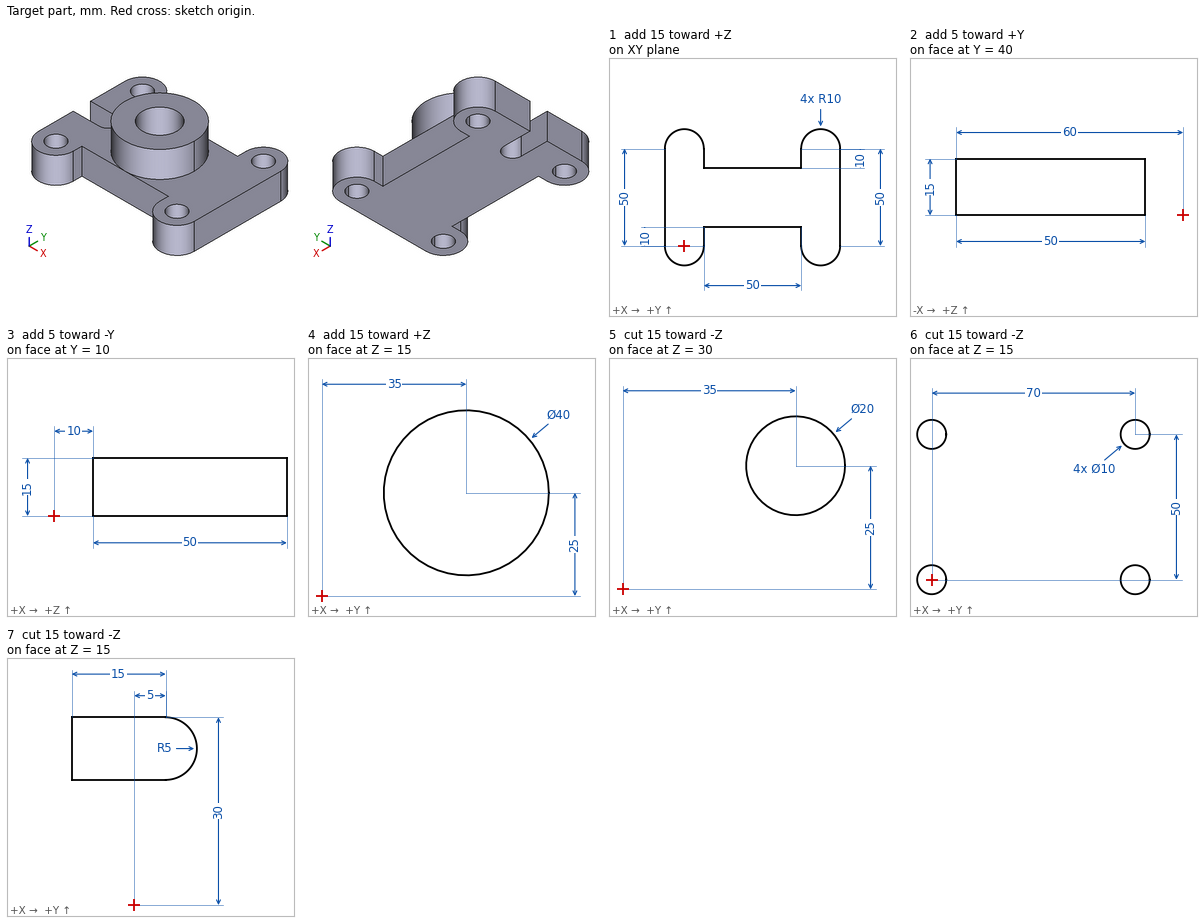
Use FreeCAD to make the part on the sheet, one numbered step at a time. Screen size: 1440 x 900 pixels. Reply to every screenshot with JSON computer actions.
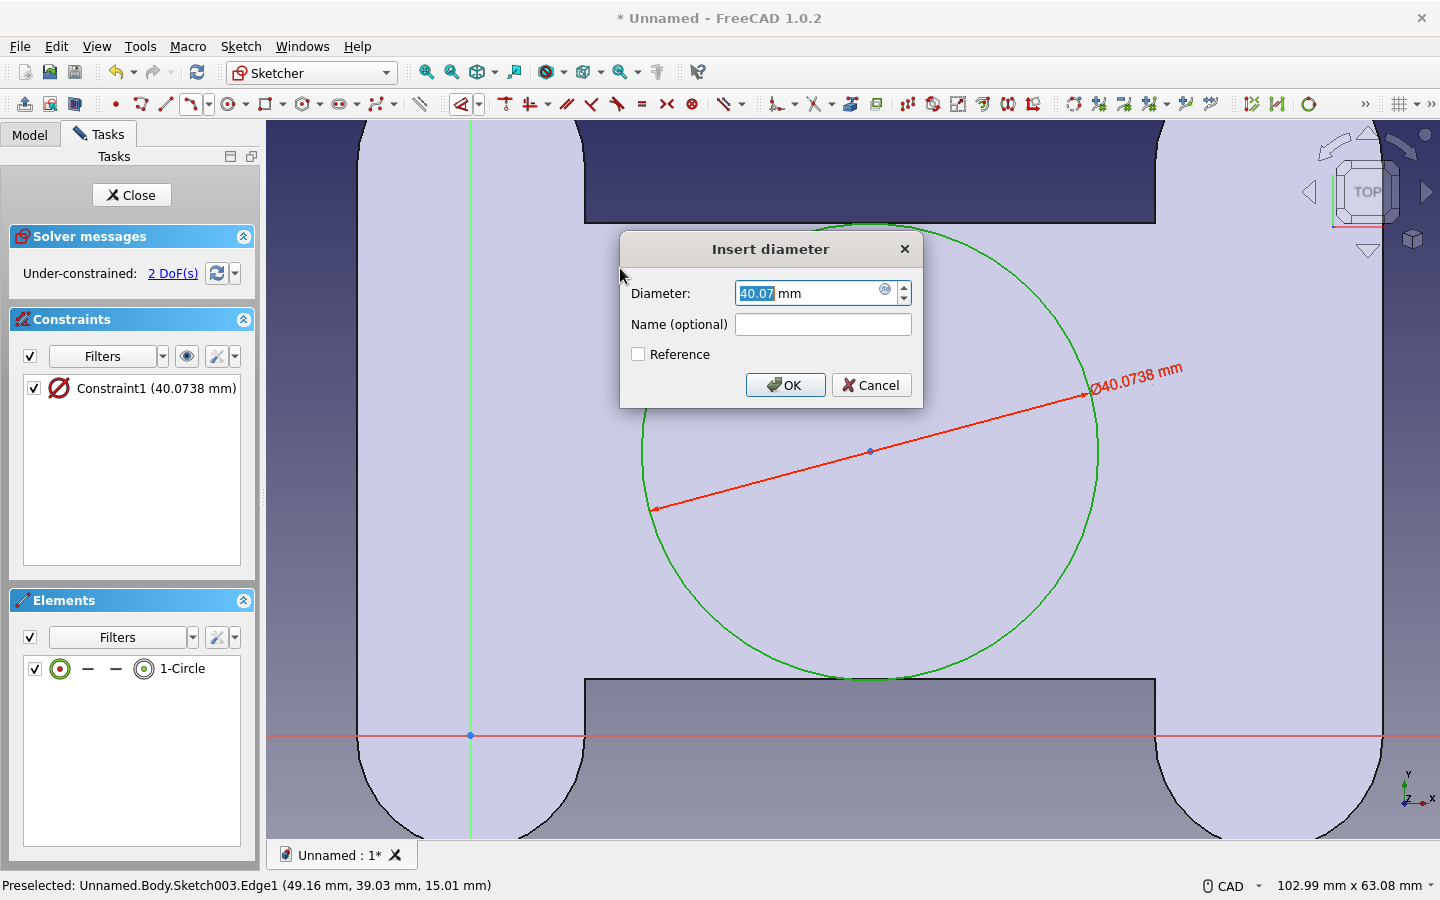
{"action": "type", "text": "40"}
{"action": "key", "text": "Return"}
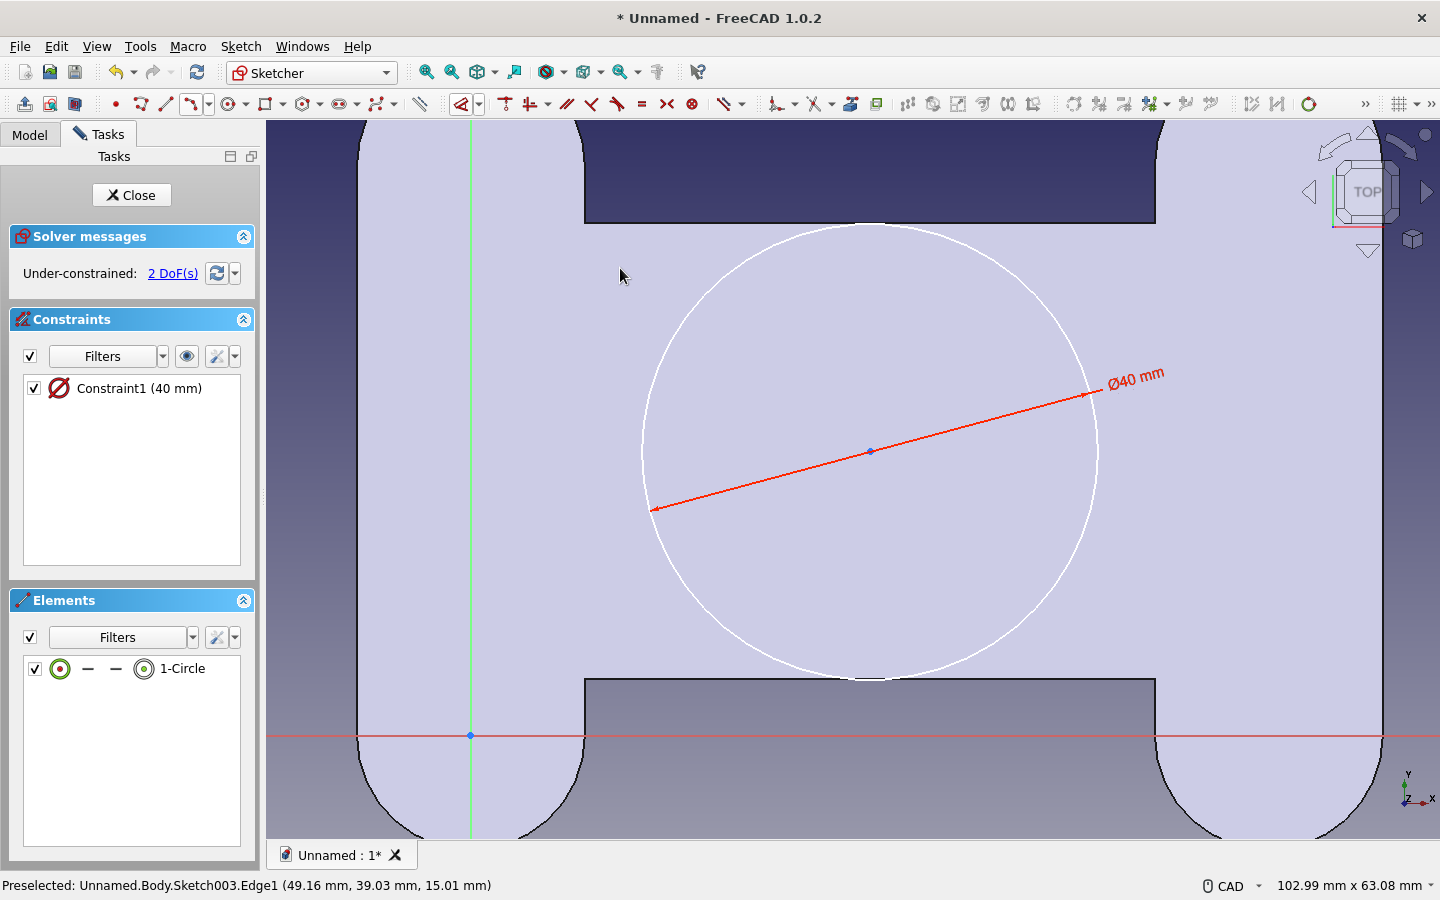
{"action": "left_click", "coordinate": [870, 452]}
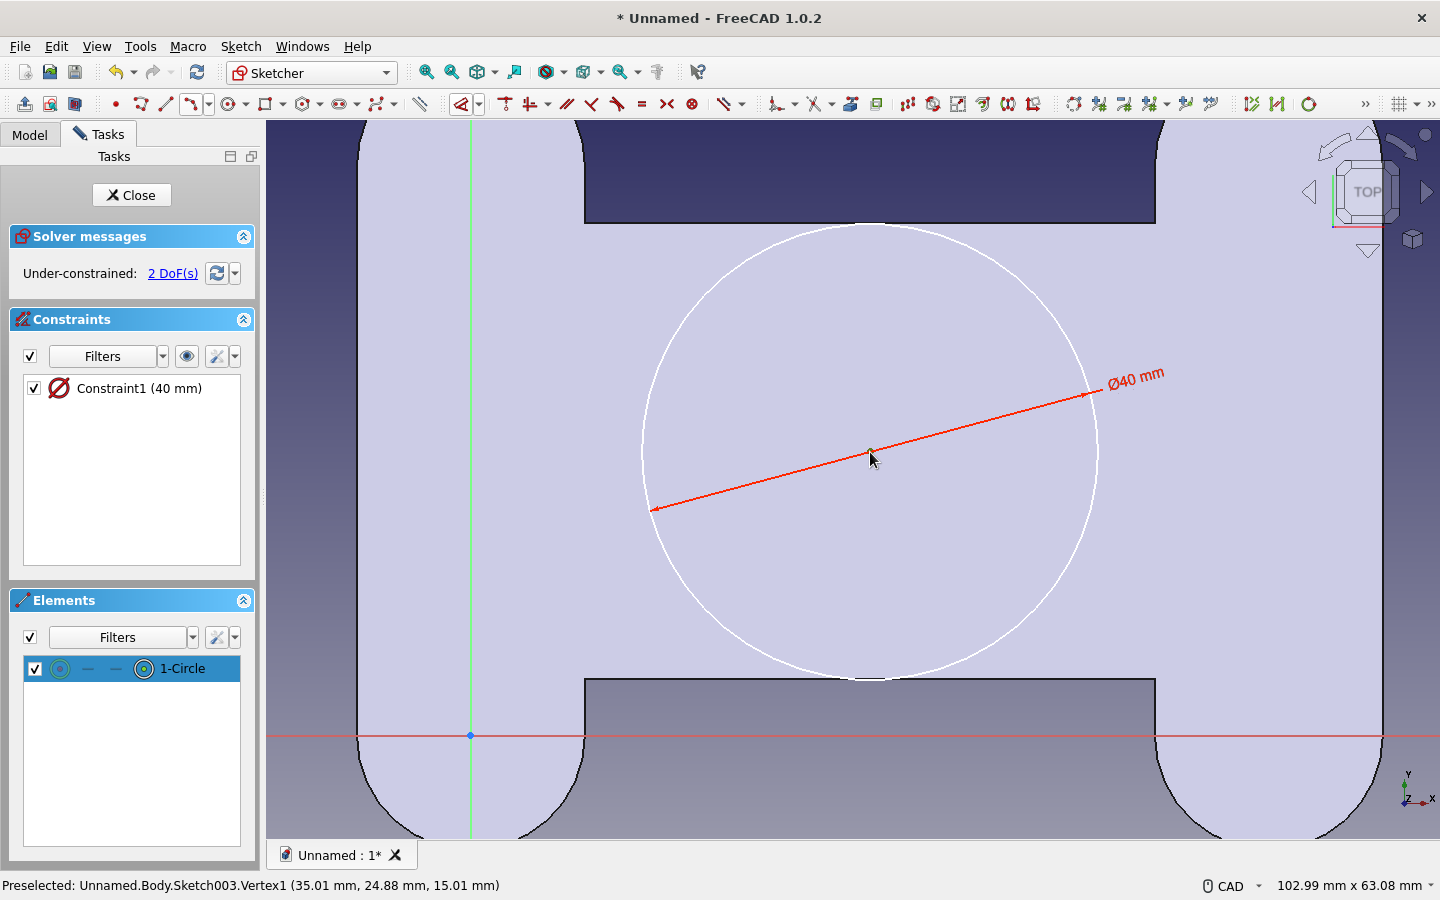
{"action": "left_click", "coordinate": [478, 104]}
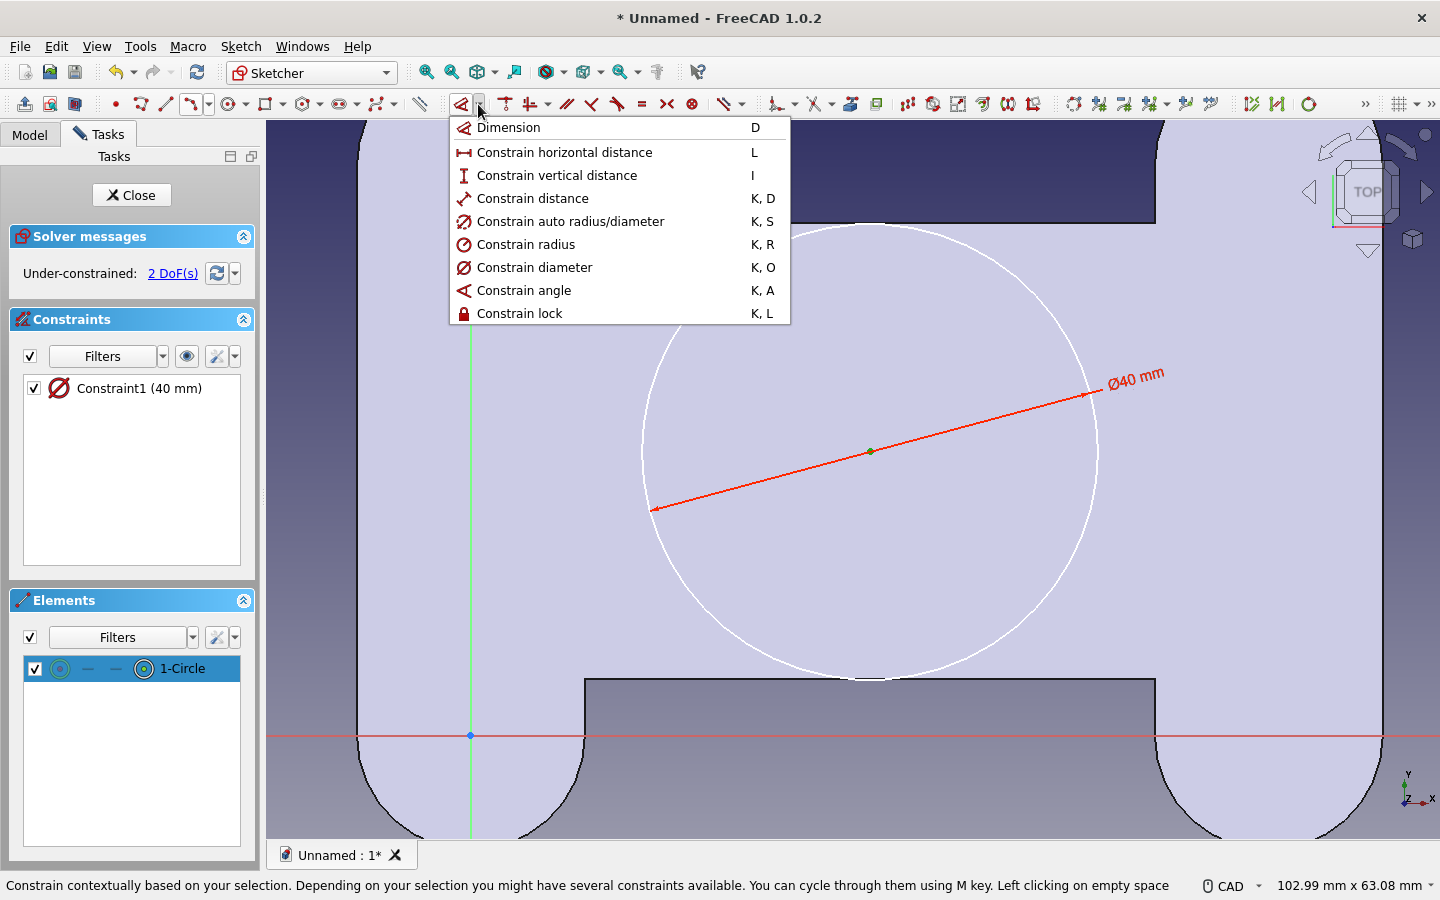
{"action": "left_click", "coordinate": [620, 152]}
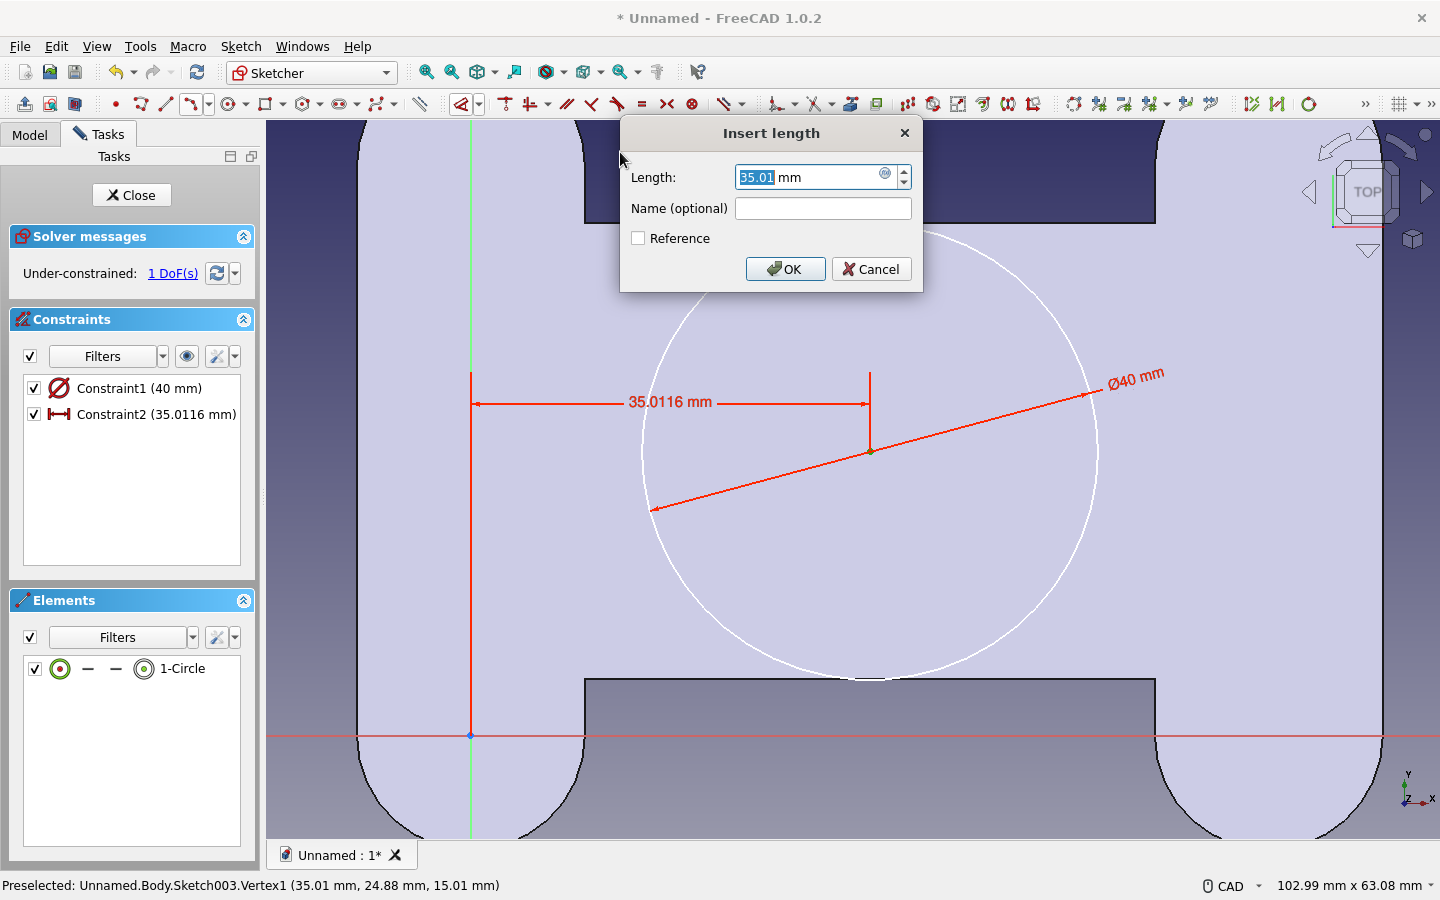
{"action": "type", "text": "35"}
{"action": "key", "text": "Return"}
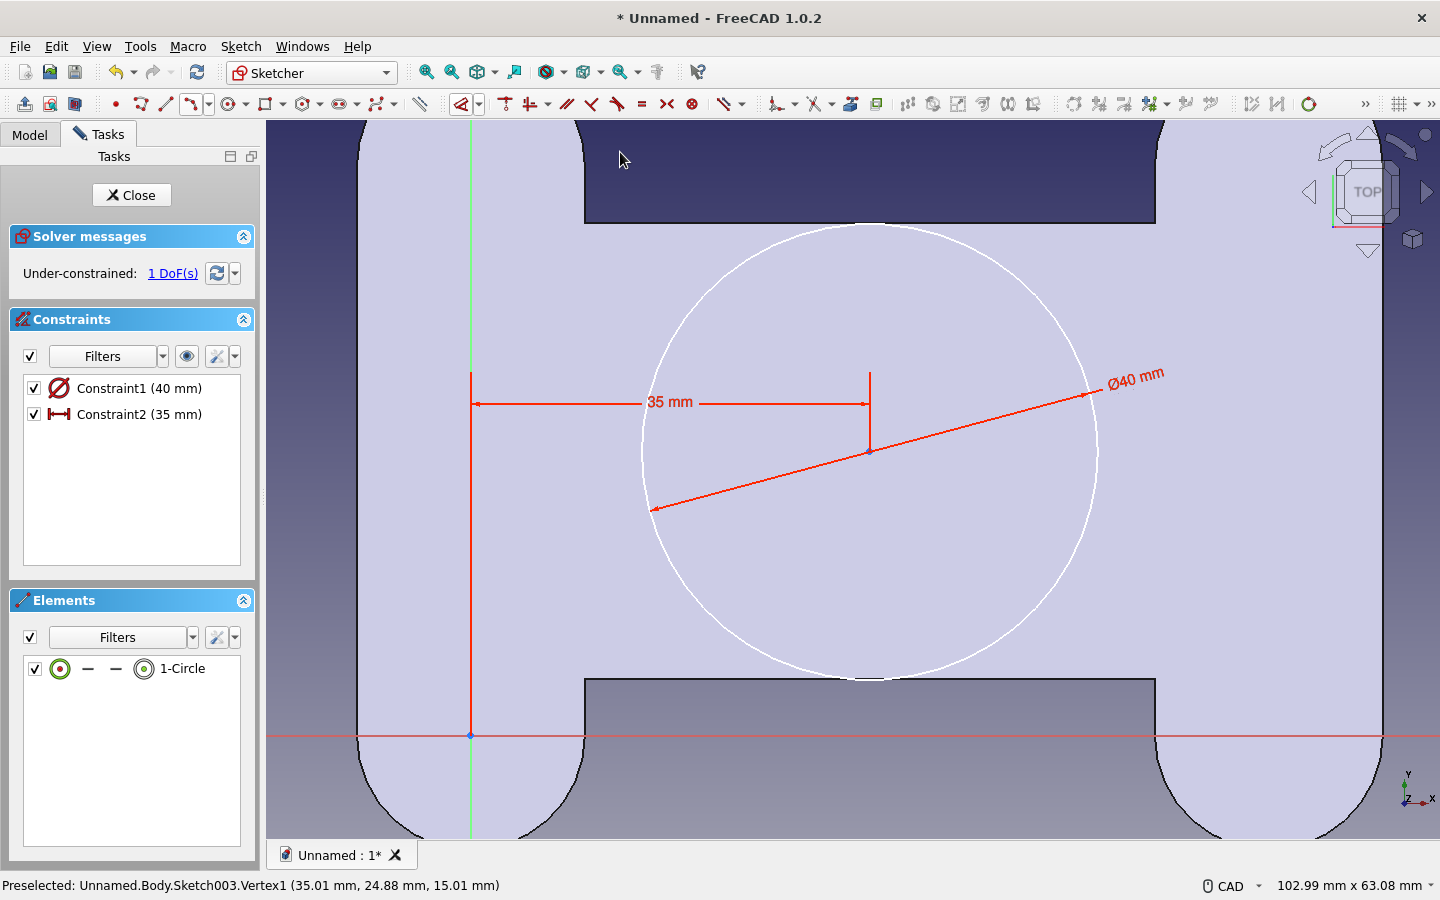
{"action": "left_click", "coordinate": [870, 452]}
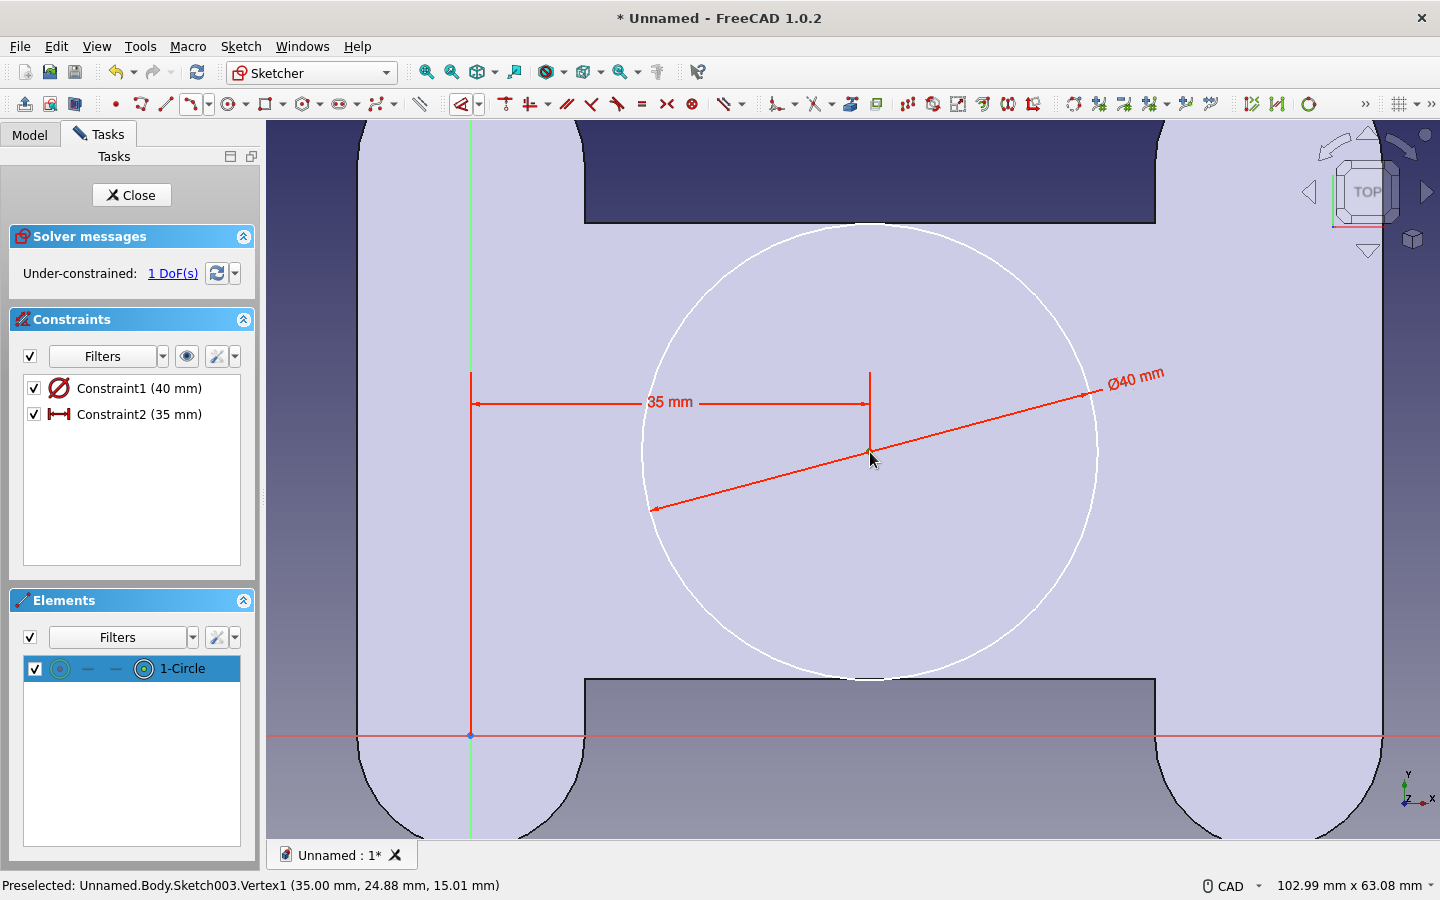
{"action": "left_click", "coordinate": [478, 104]}